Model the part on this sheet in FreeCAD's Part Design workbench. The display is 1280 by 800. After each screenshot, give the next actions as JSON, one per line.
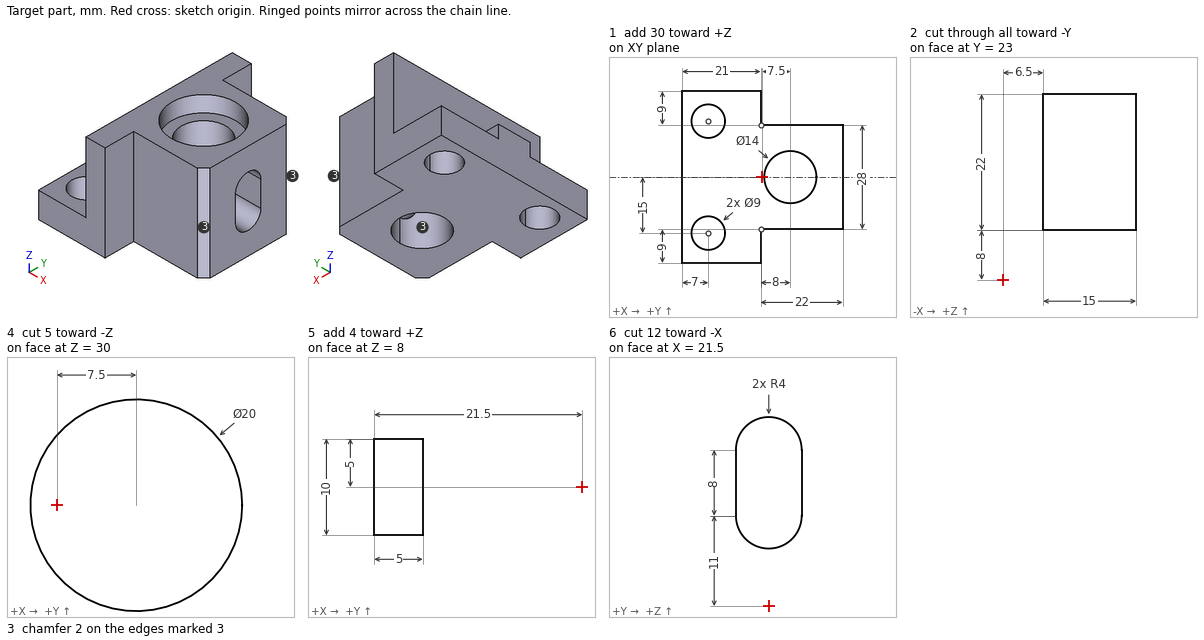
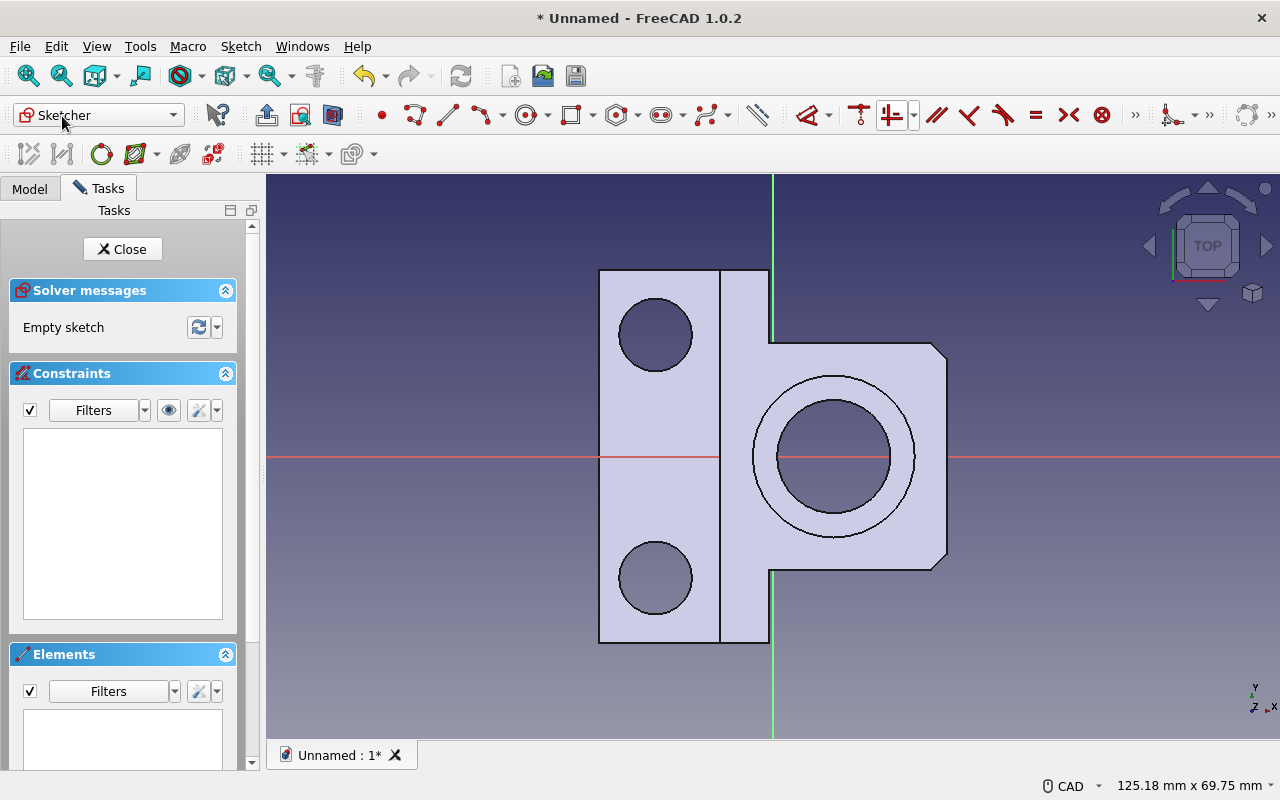
{"action": "key", "text": "q s"}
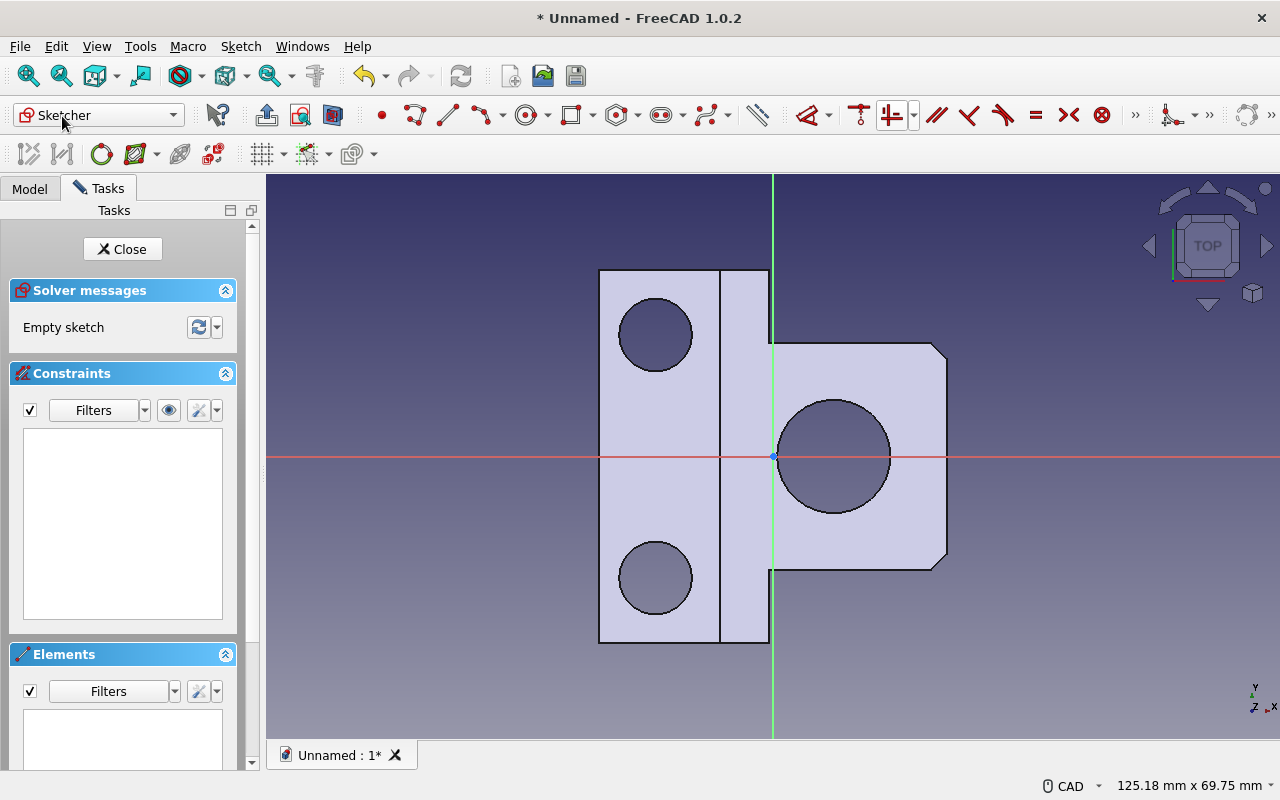
{"action": "scroll", "coordinate": [678, 456], "scroll_direction": "up", "scroll_amount": 6}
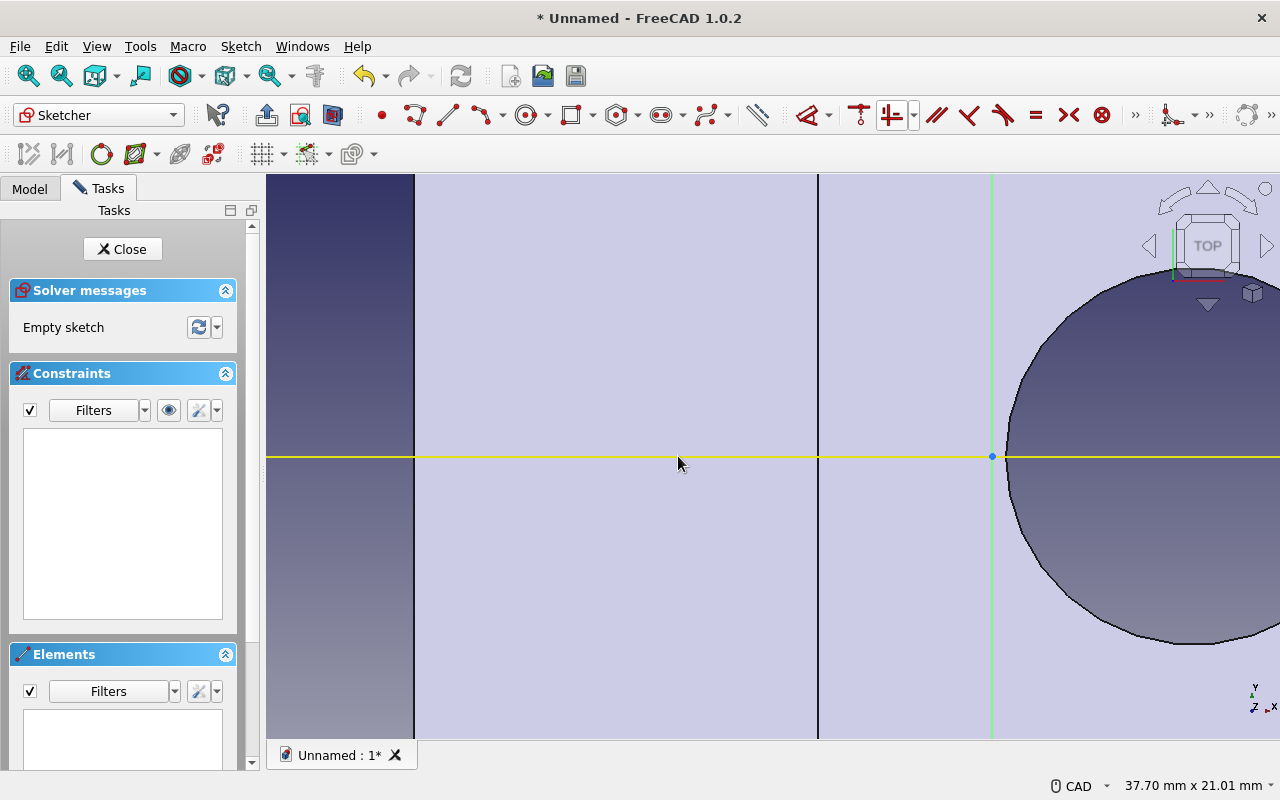
{"action": "key", "text": "g r"}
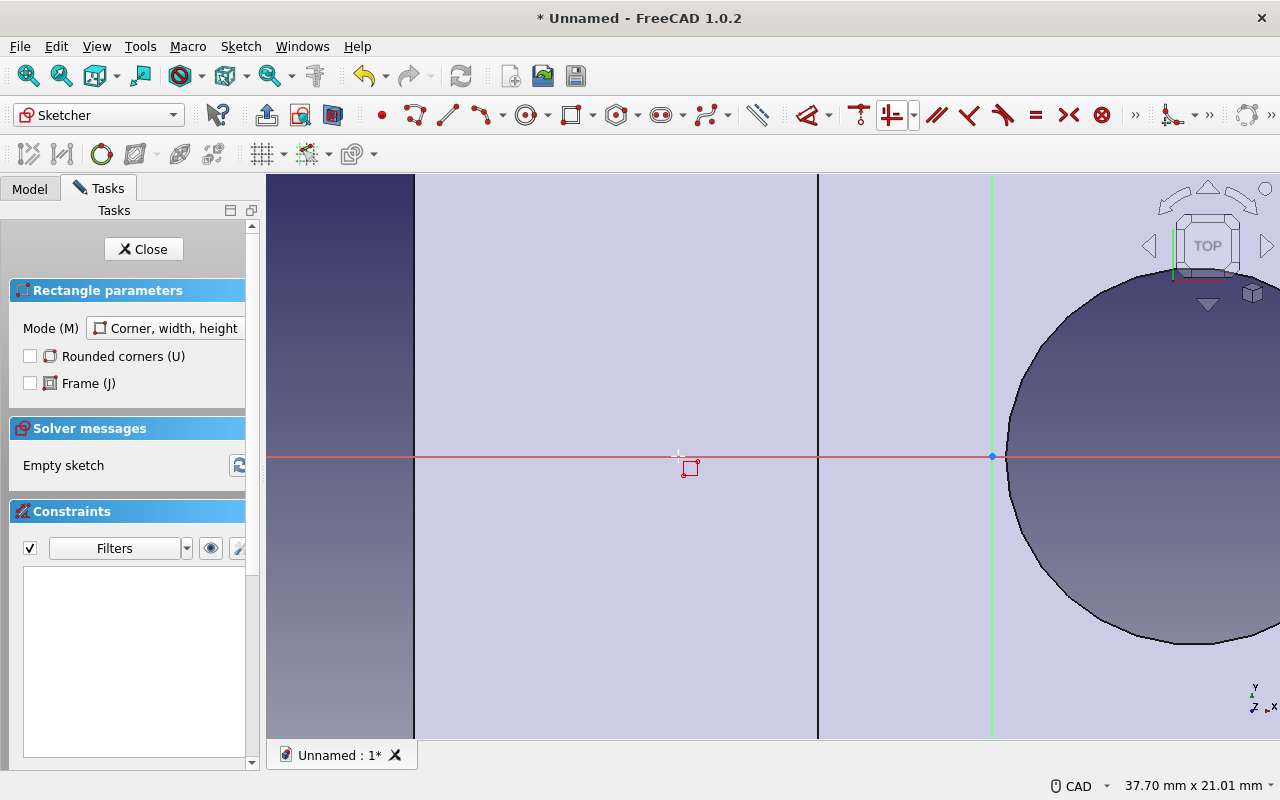
{"action": "left_click", "coordinate": [414, 322]}
{"action": "left_click", "coordinate": [549, 591]}
{"action": "key", "text": "Escape"}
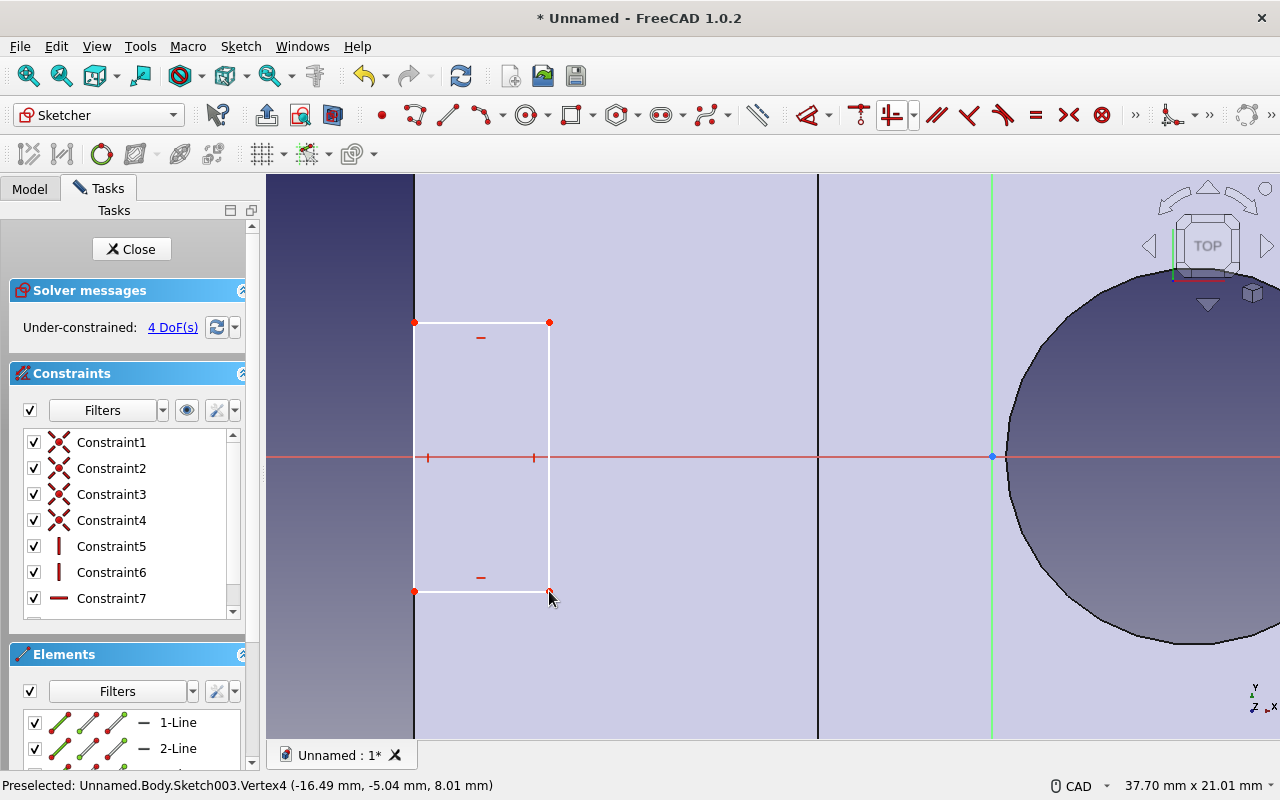
{"action": "key", "text": "d"}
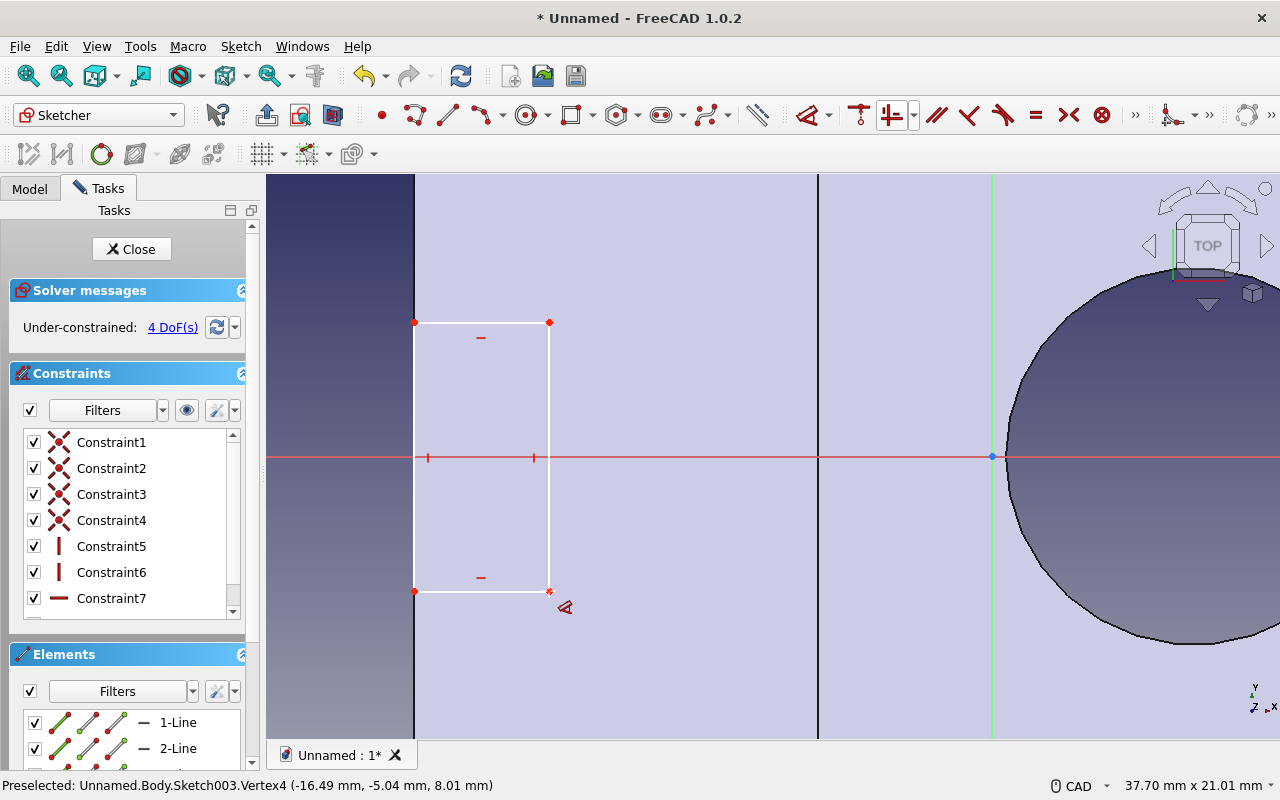
{"action": "left_click", "coordinate": [455, 592]}
{"action": "left_click", "coordinate": [482, 626]}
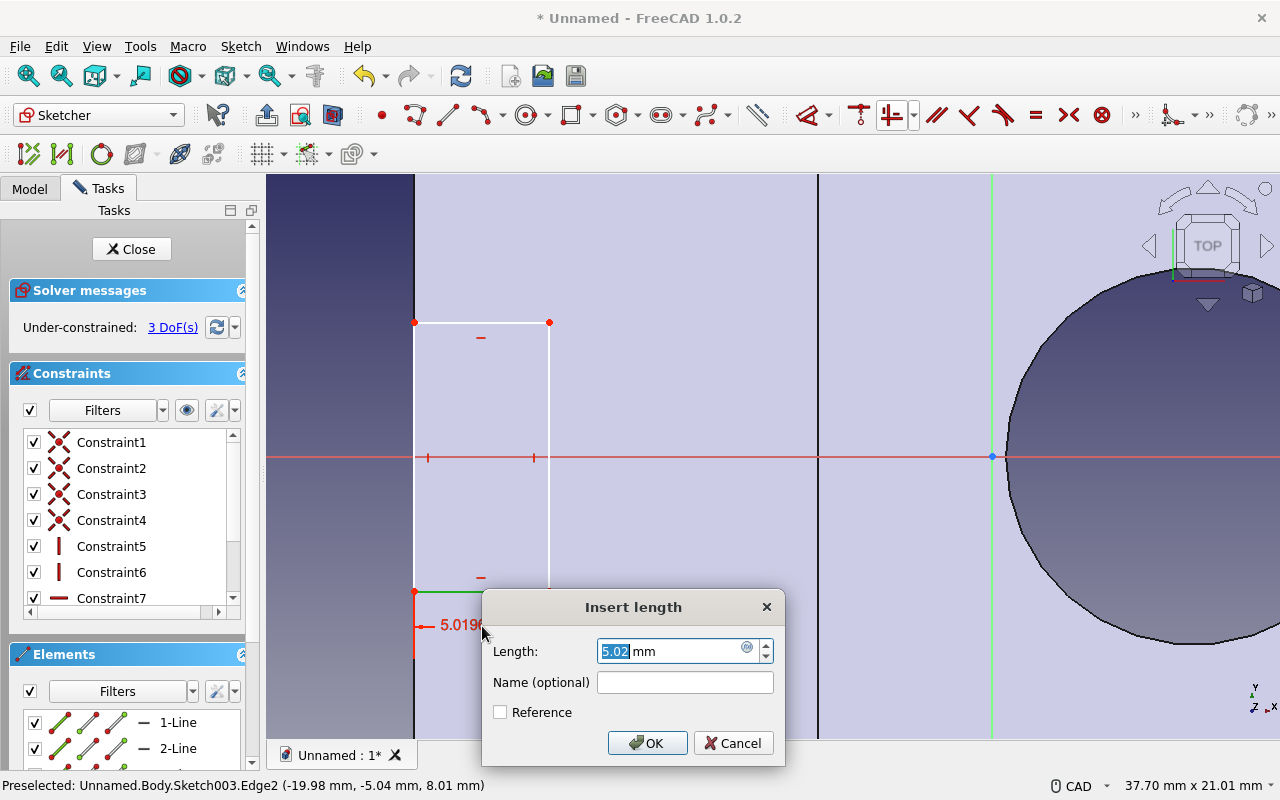
{"action": "type", "text": "5"}
{"action": "key", "text": "Return"}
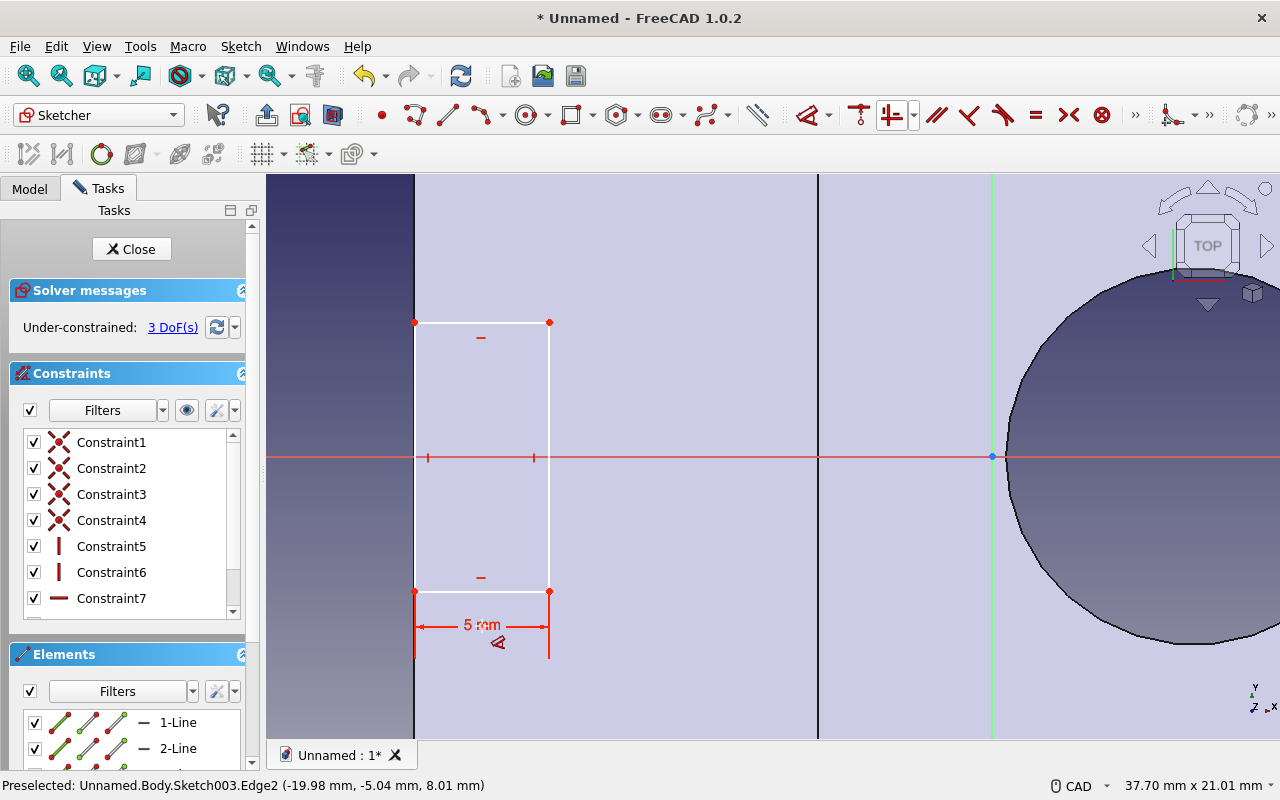
{"action": "left_click", "coordinate": [415, 404]}
{"action": "left_click", "coordinate": [381, 396]}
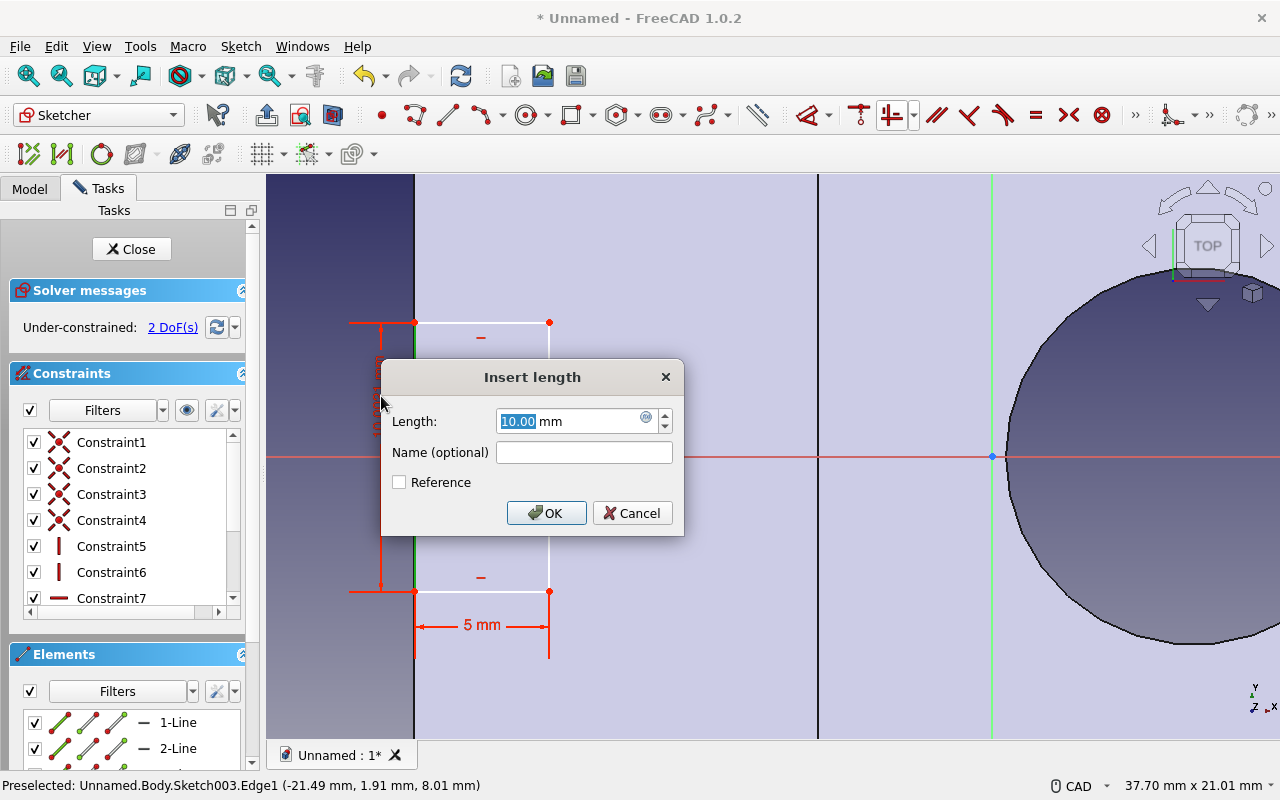
{"action": "type", "text": "10"}
{"action": "key", "text": "Return"}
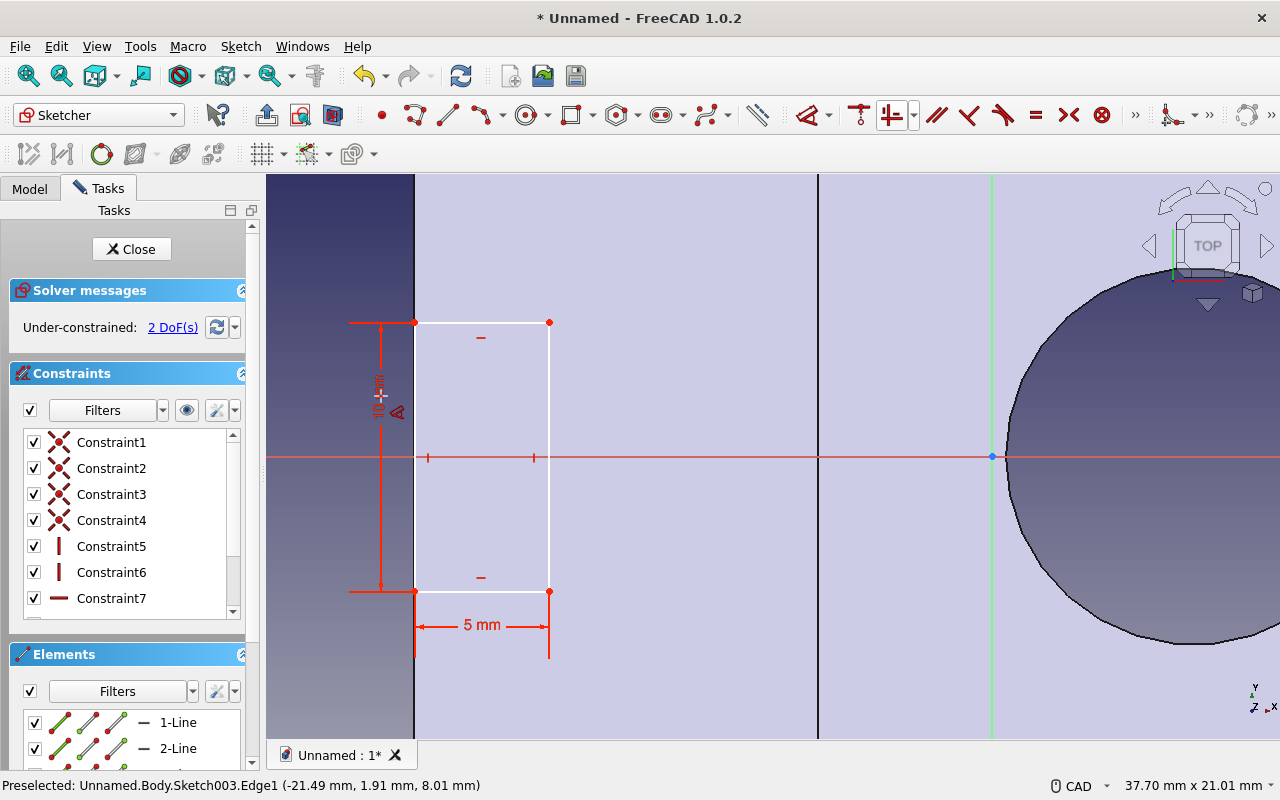
{"action": "left_click", "coordinate": [415, 323]}
{"action": "left_click", "coordinate": [1026, 390]}